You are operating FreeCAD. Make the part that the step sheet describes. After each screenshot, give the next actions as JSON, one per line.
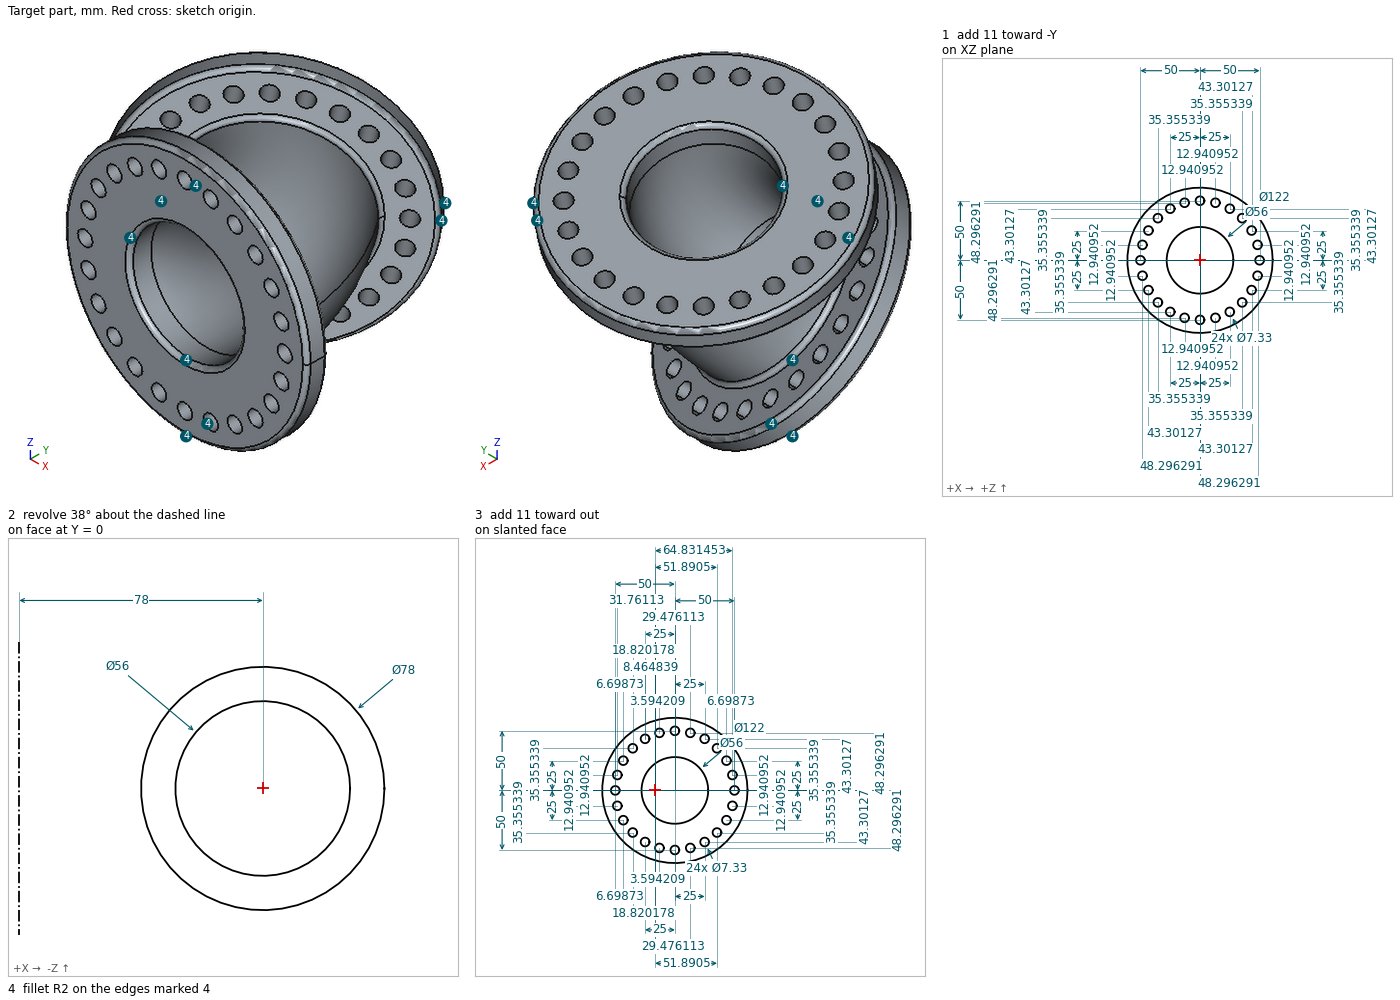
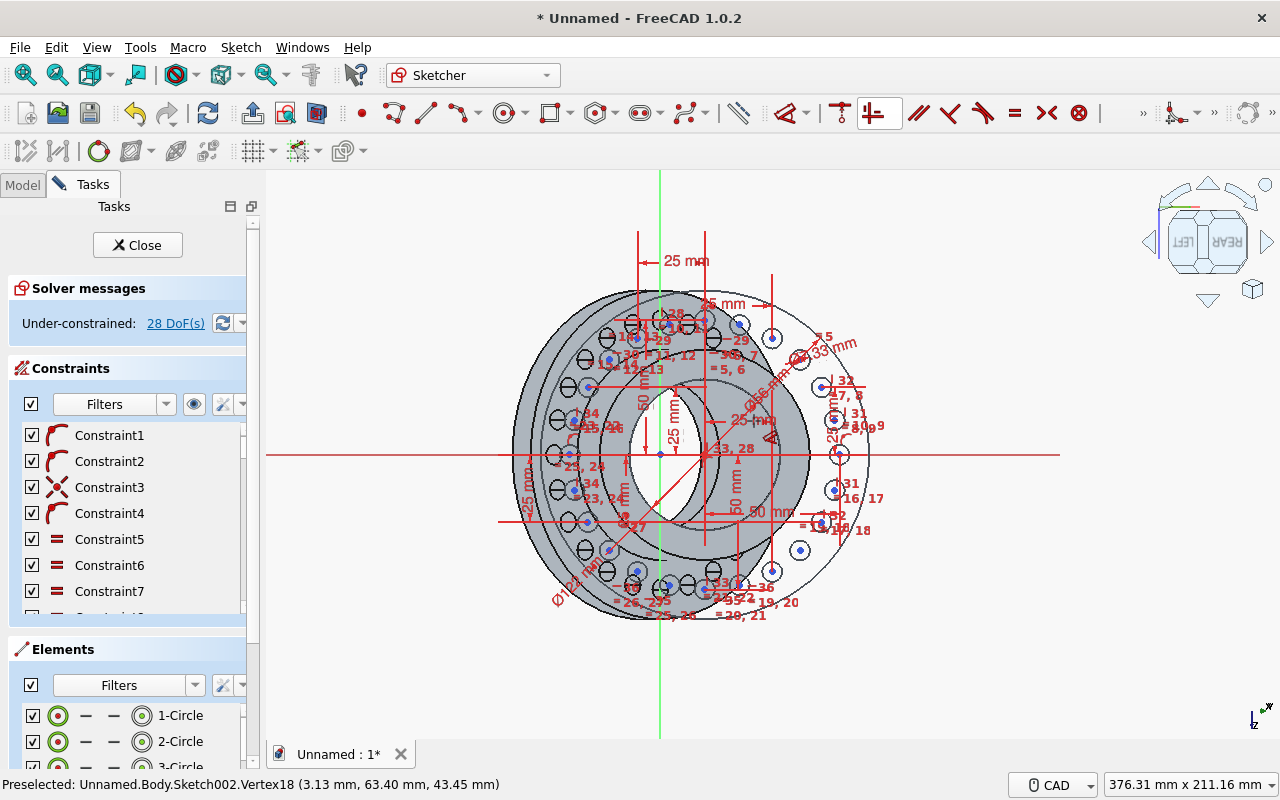
{"action": "left_click", "coordinate": [705, 455]}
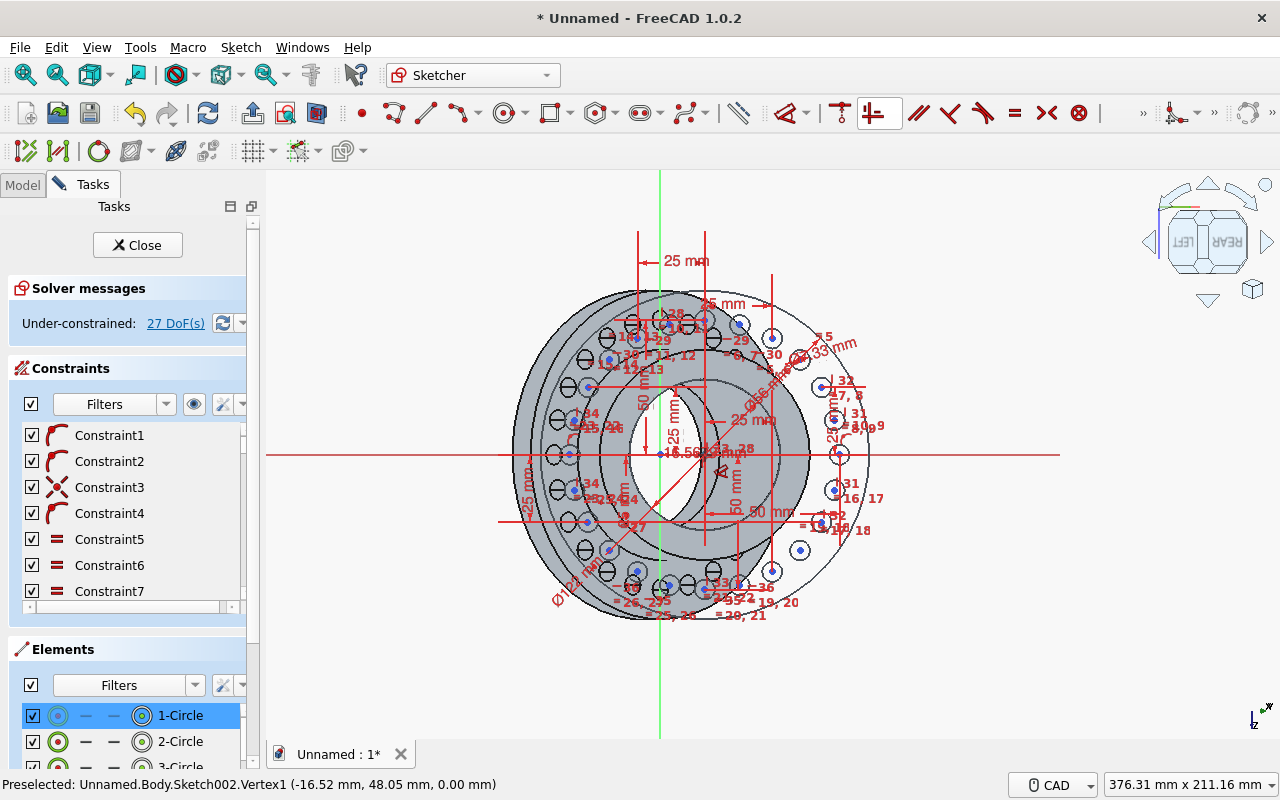
{"action": "left_click", "coordinate": [570, 455]}
{"action": "left_click", "coordinate": [637, 537]}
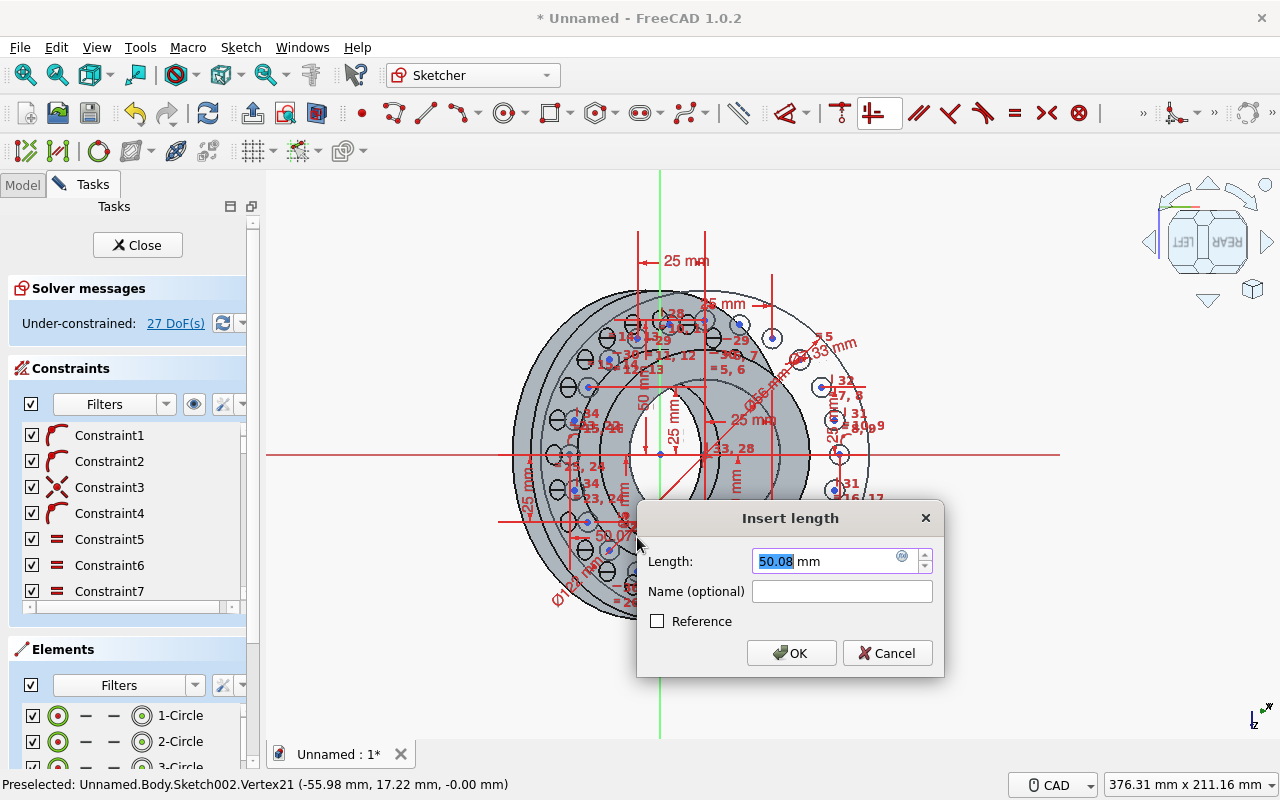
{"action": "type", "text": "50"}
{"action": "key", "text": "Return"}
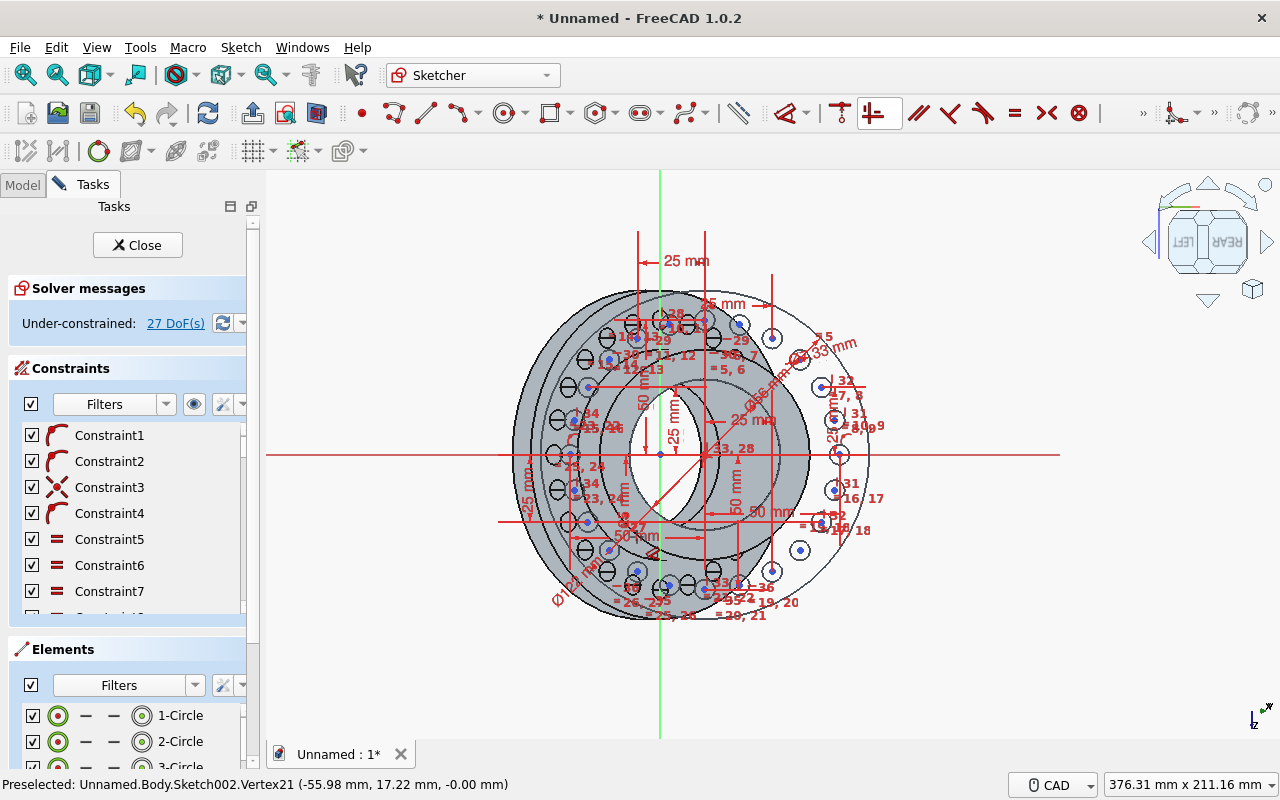
{"action": "left_click", "coordinate": [705, 590]}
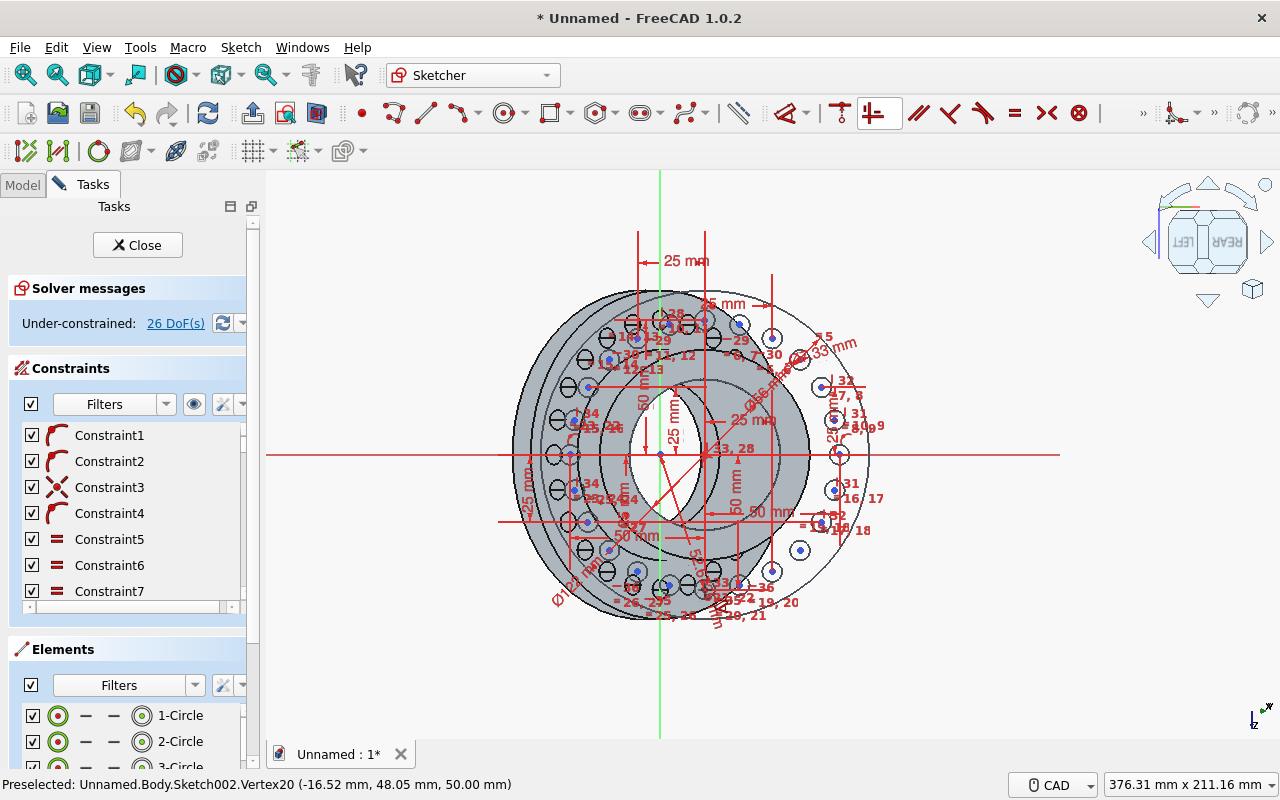
{"action": "left_click", "coordinate": [638, 572]}
{"action": "left_click", "coordinate": [687, 648]}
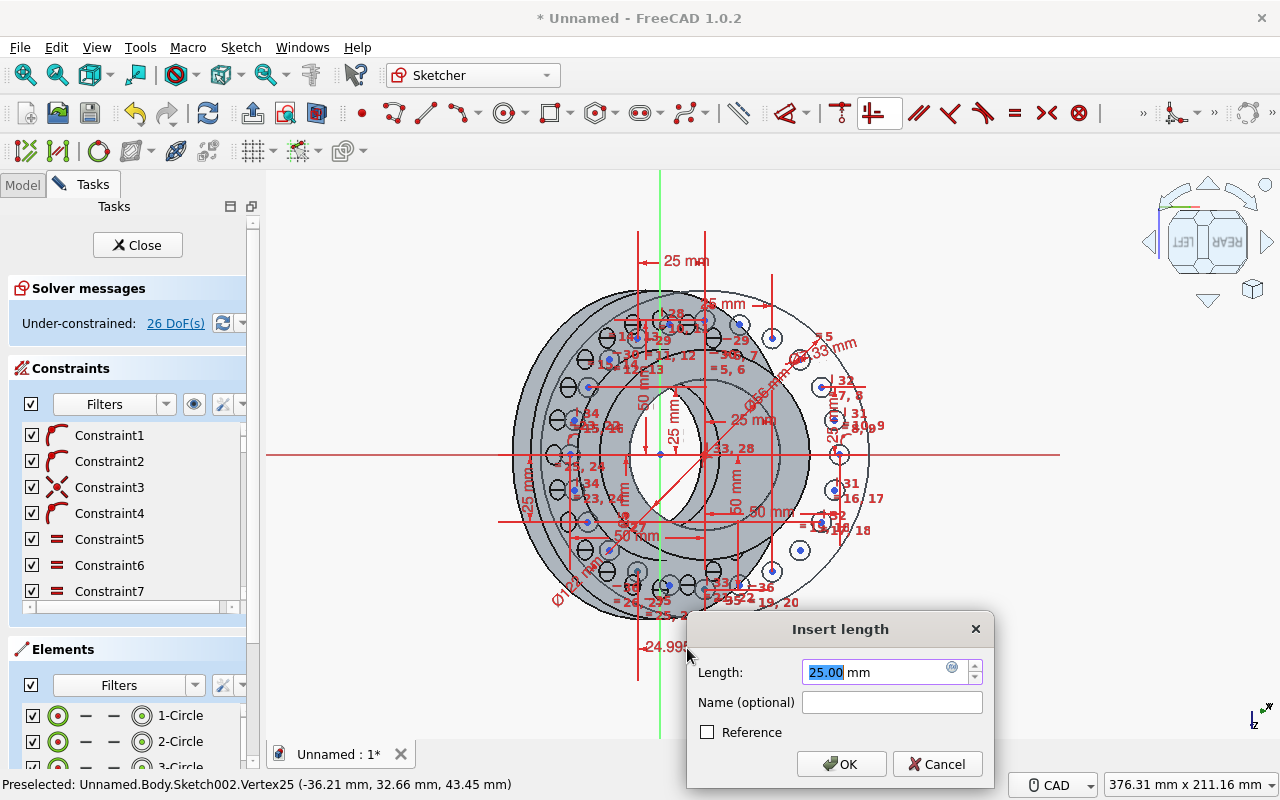
{"action": "type", "text": "25"}
{"action": "key", "text": "Return"}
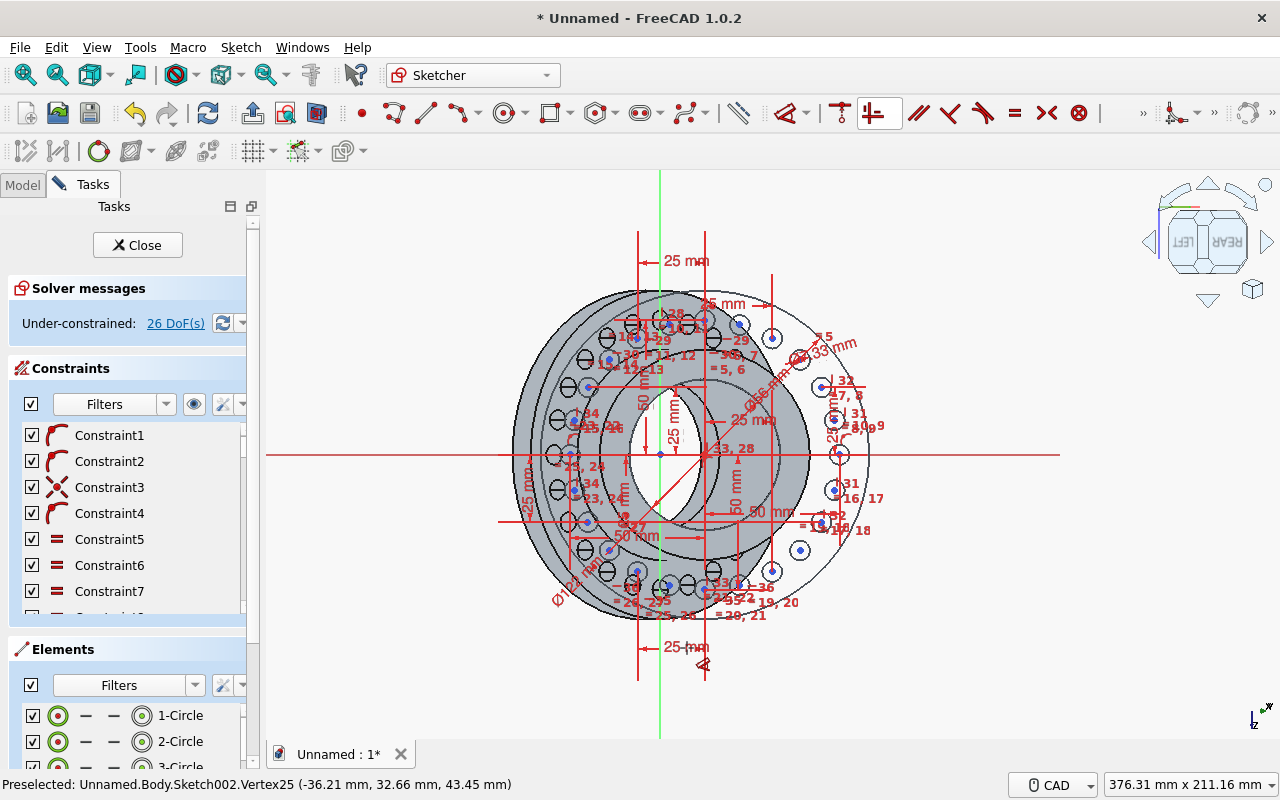
{"action": "left_click", "coordinate": [800, 360]}
{"action": "left_click", "coordinate": [698, 513]}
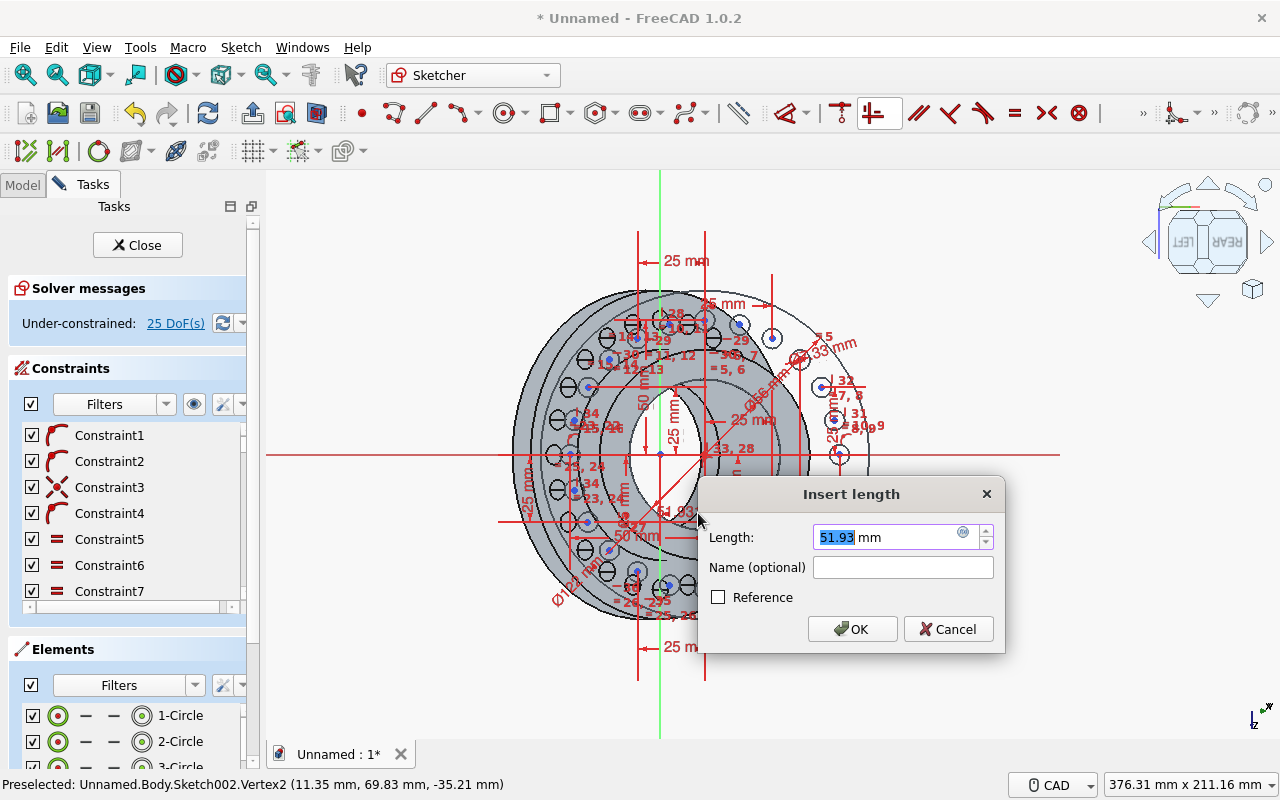
{"action": "type", "text": "51.8905"}
{"action": "key", "text": "Return"}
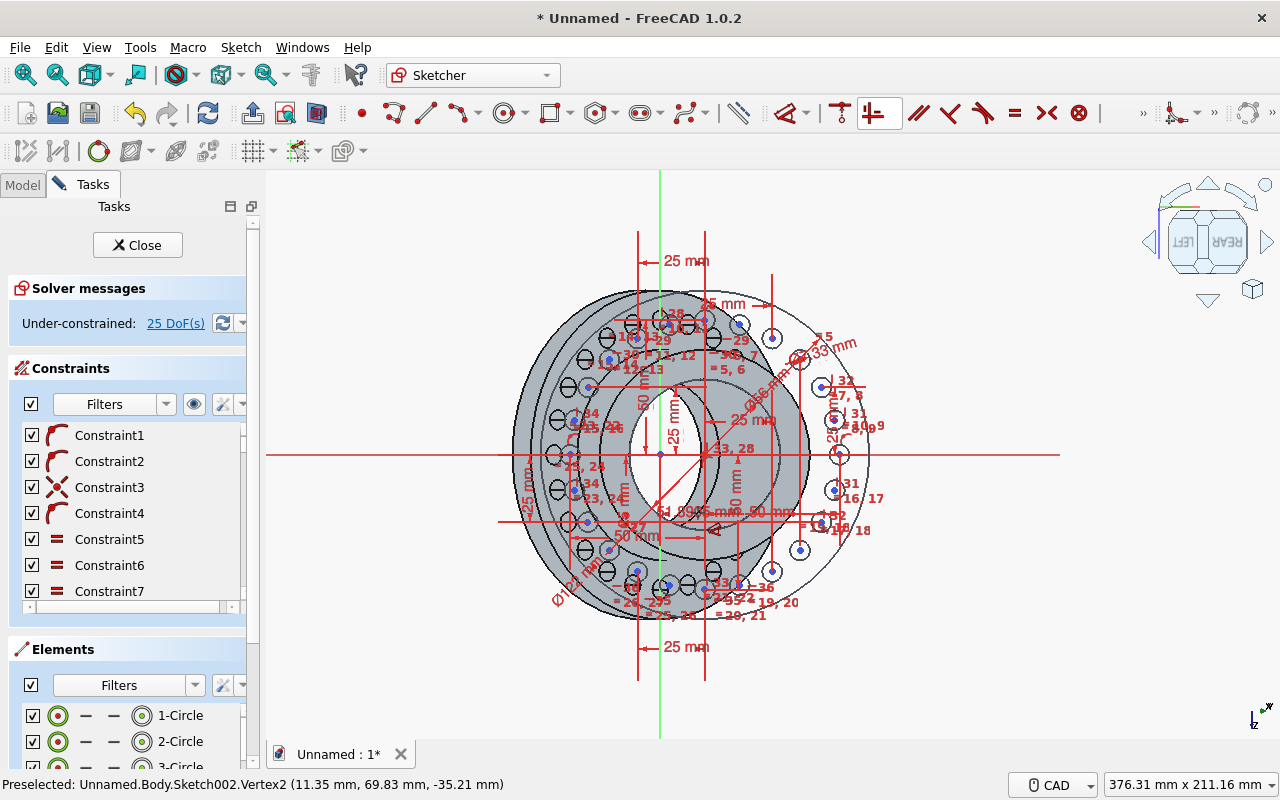
{"action": "left_click", "coordinate": [800, 551]}
{"action": "left_click", "coordinate": [762, 633]}